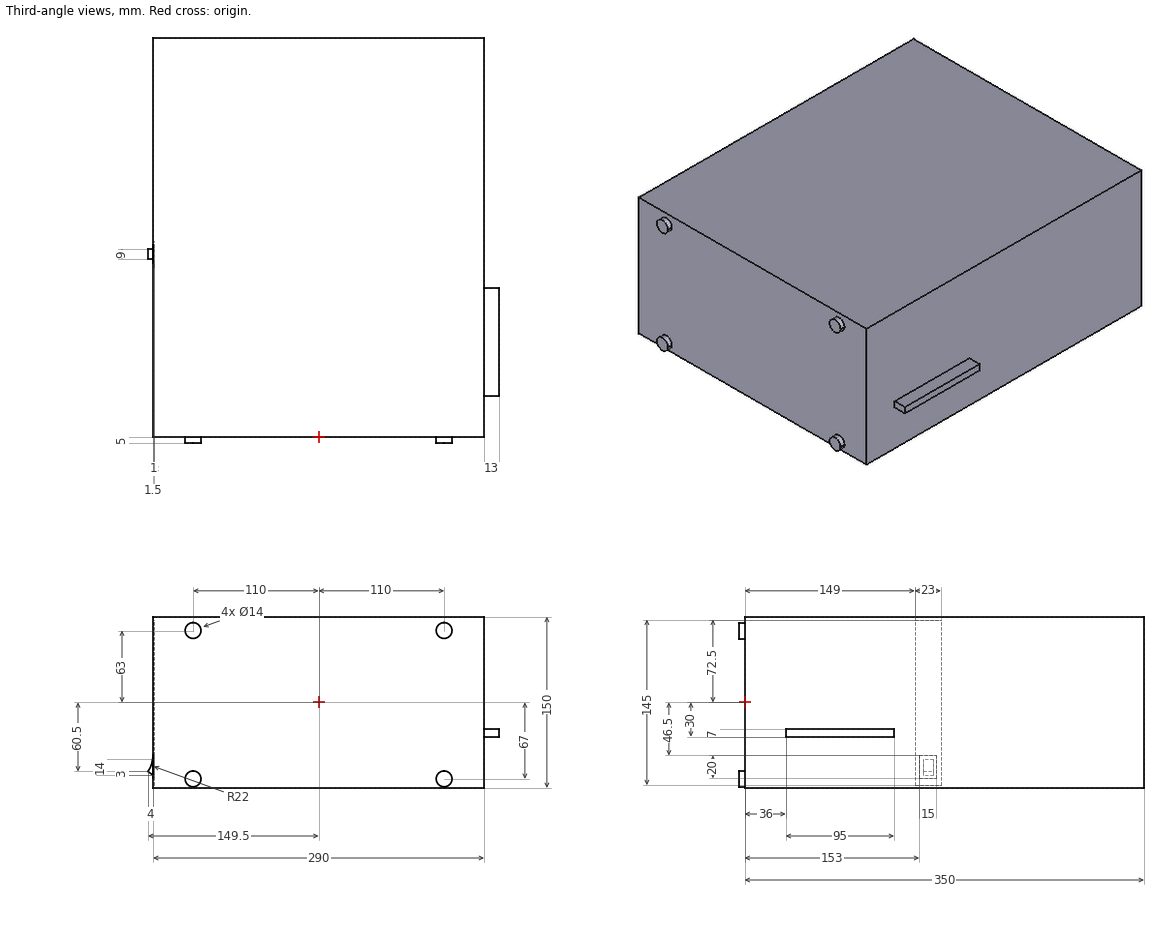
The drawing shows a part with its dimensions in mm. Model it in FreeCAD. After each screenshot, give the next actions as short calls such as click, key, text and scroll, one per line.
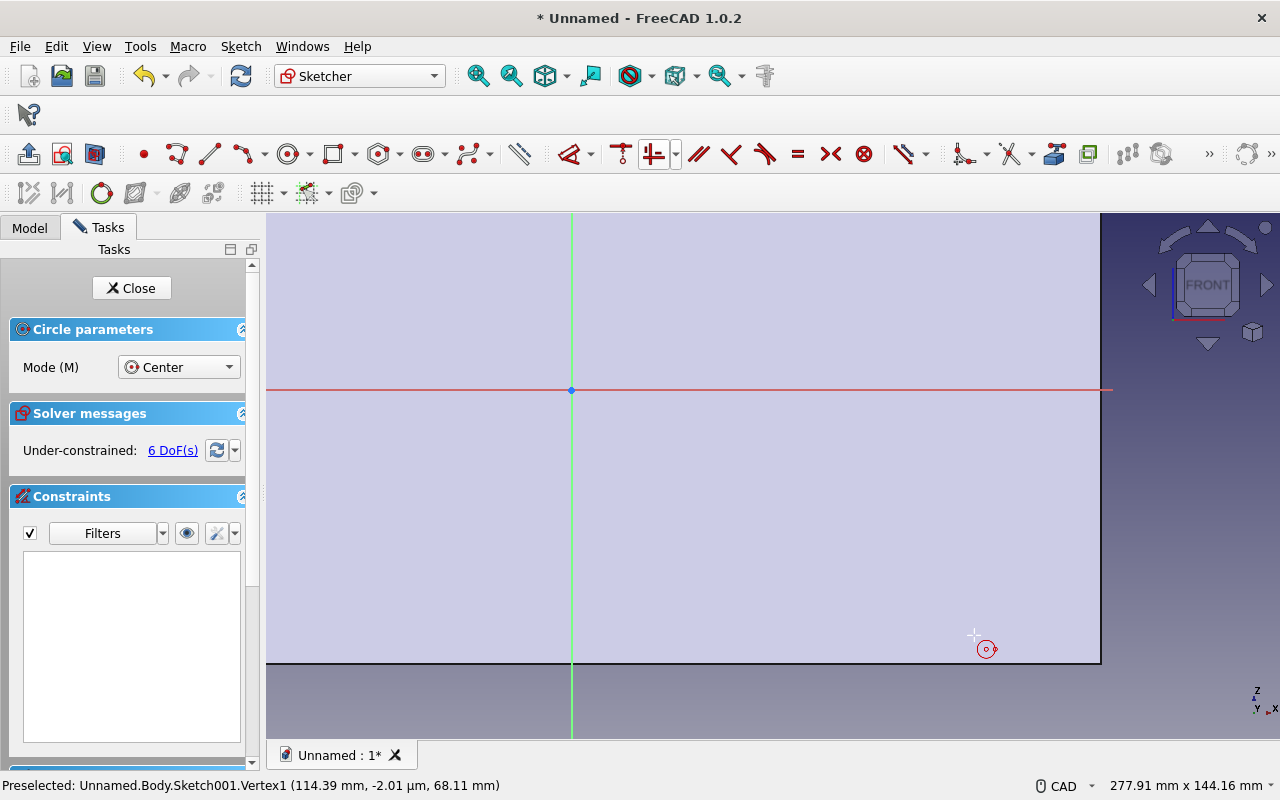
click(973, 635)
click(991, 617)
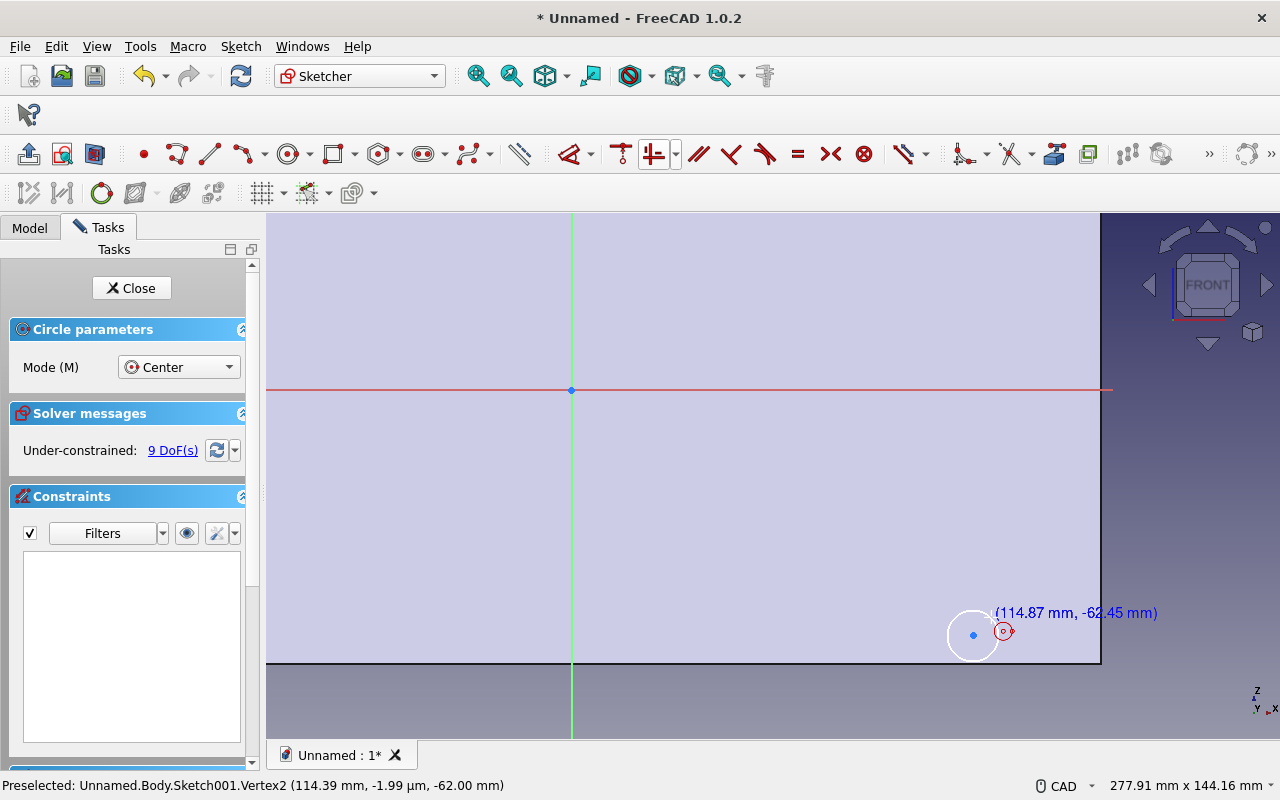
scroll(974, 636, down, 2)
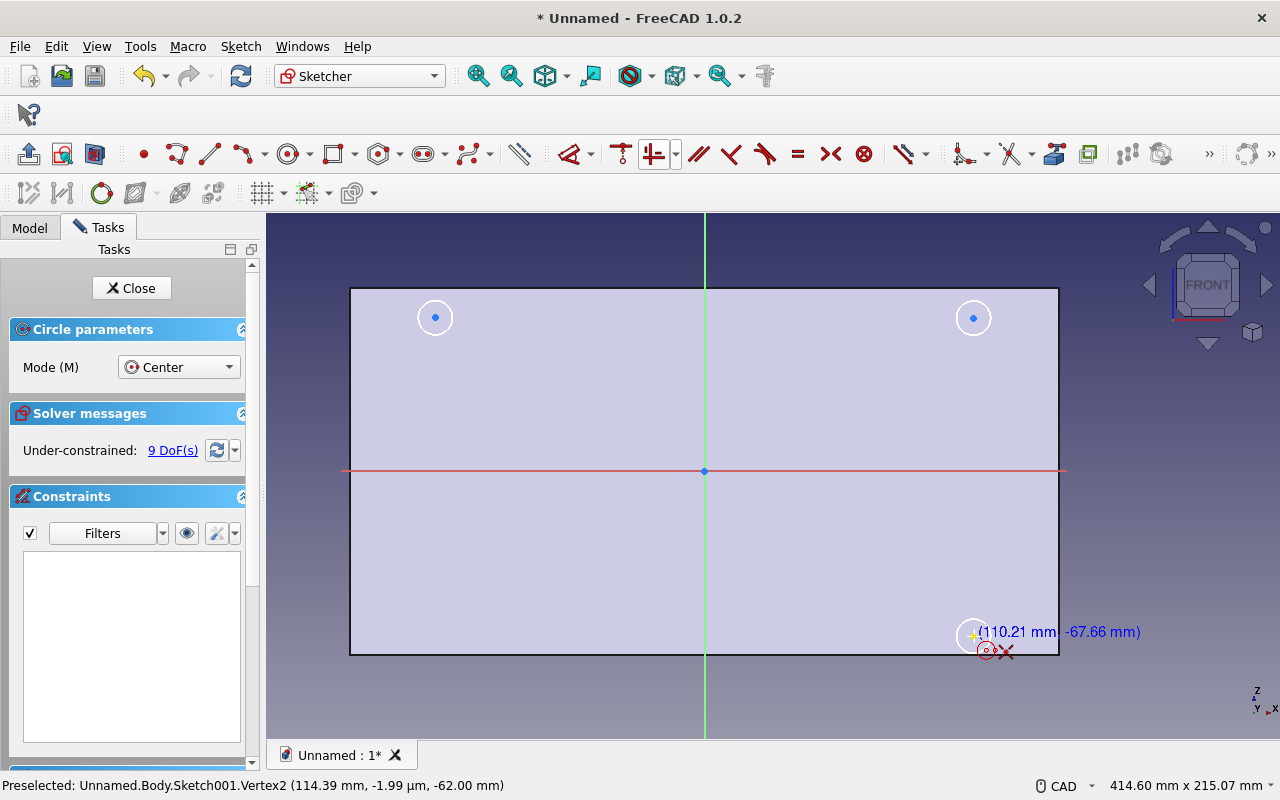
scroll(436, 635, up, 2)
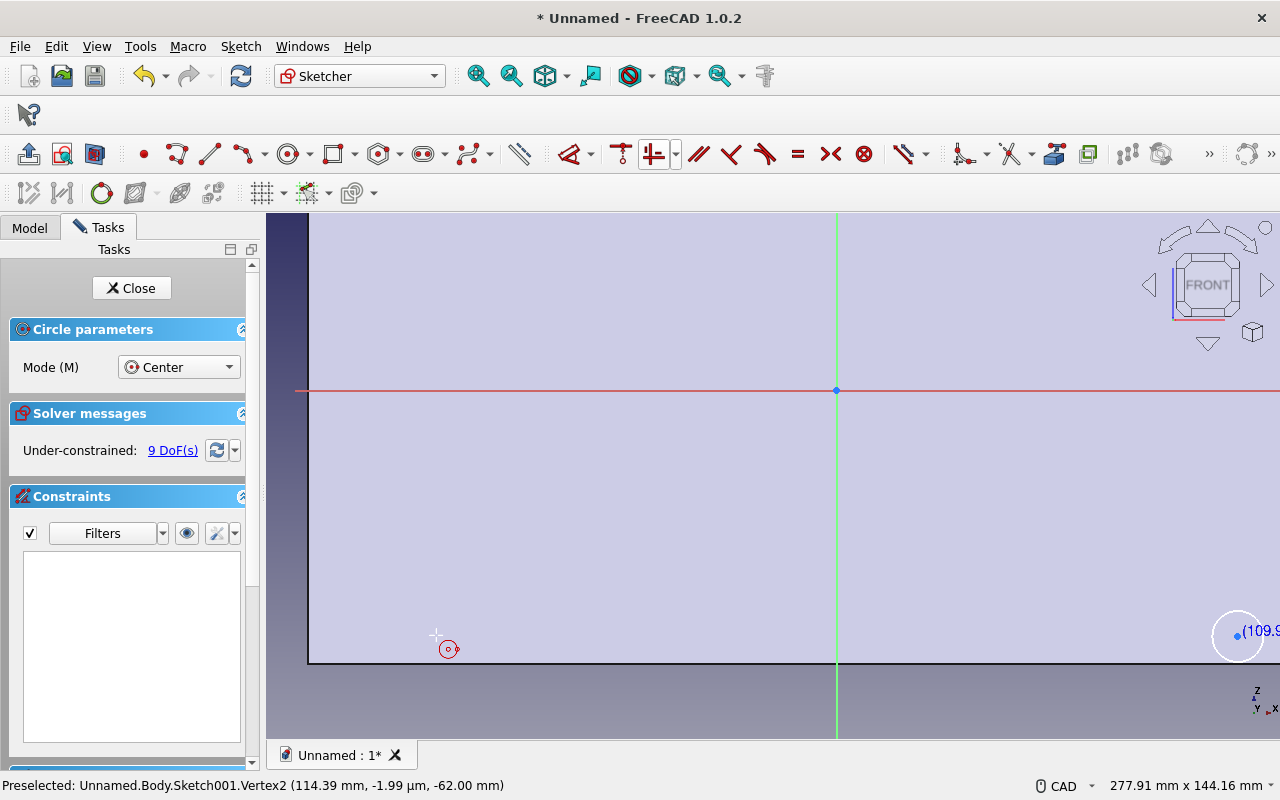
click(435, 635)
click(453, 617)
key(Escape)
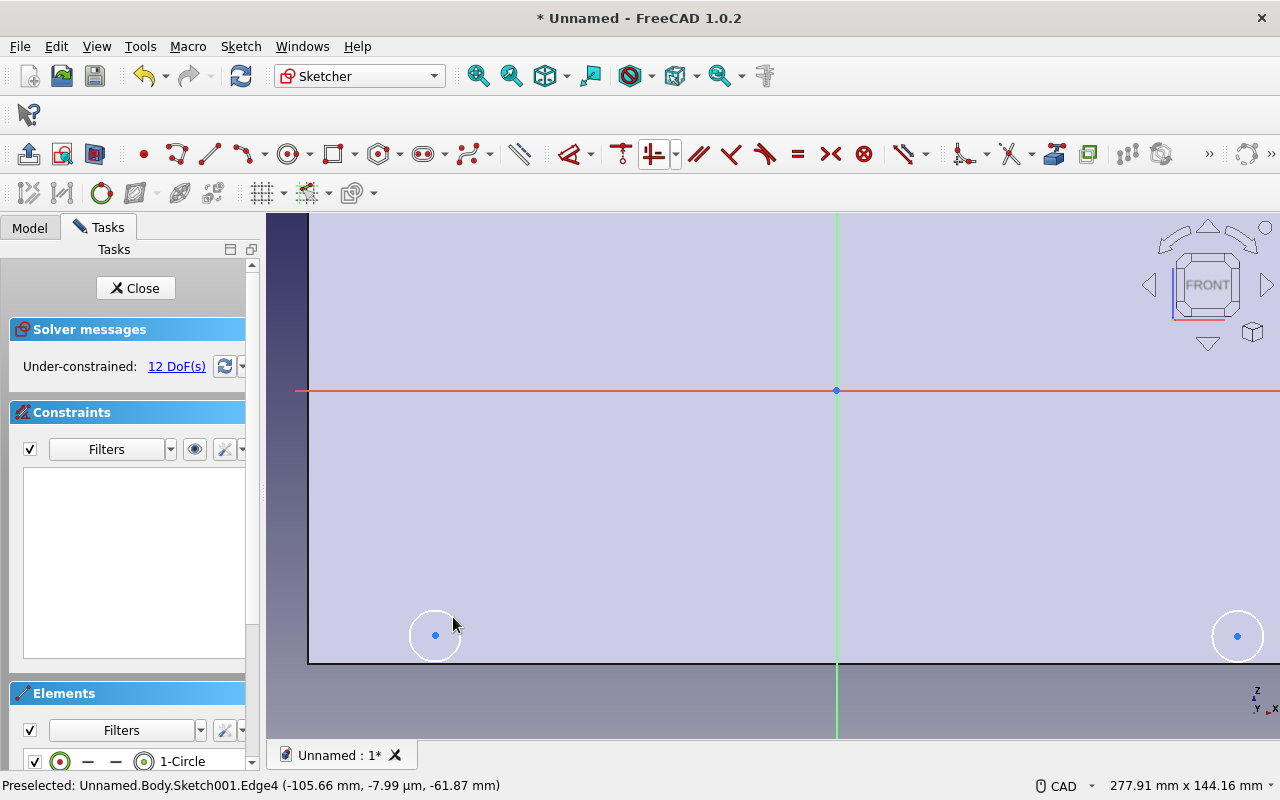
scroll(436, 635, down, 2)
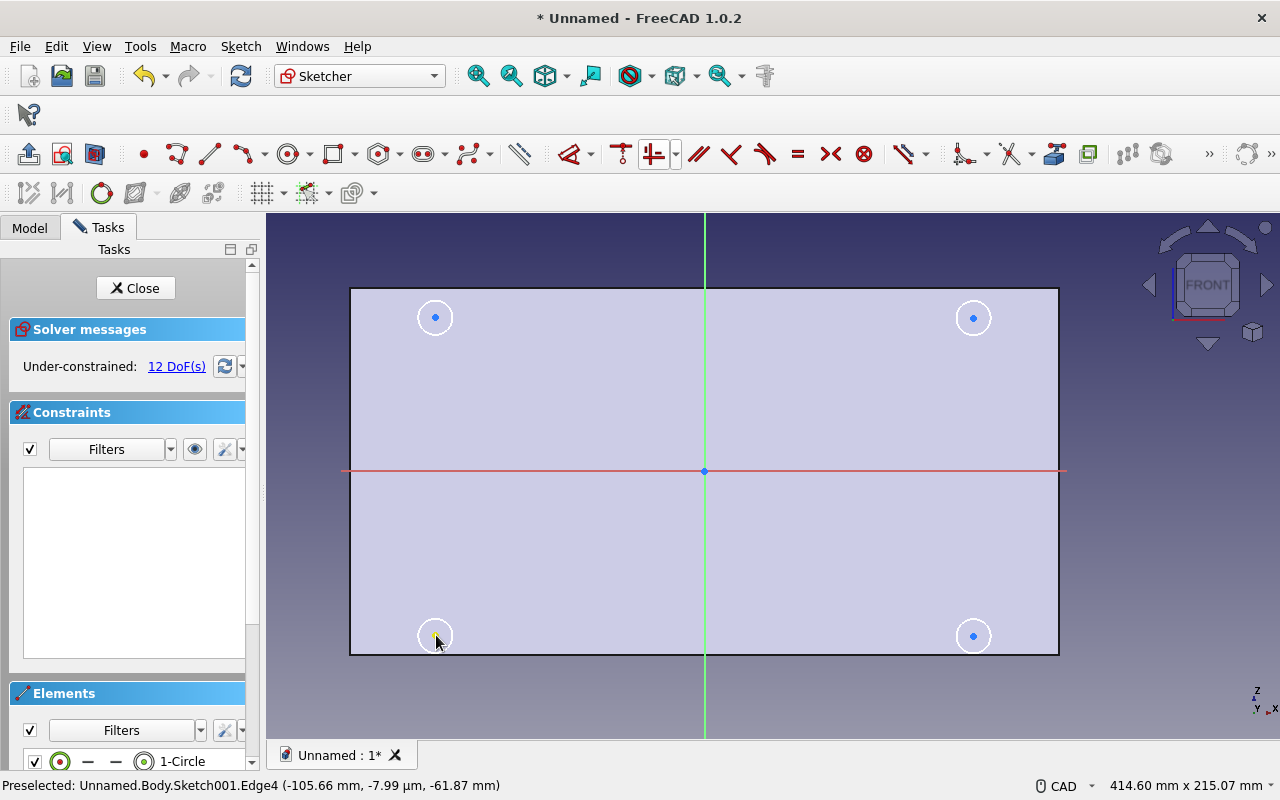
click(447, 306)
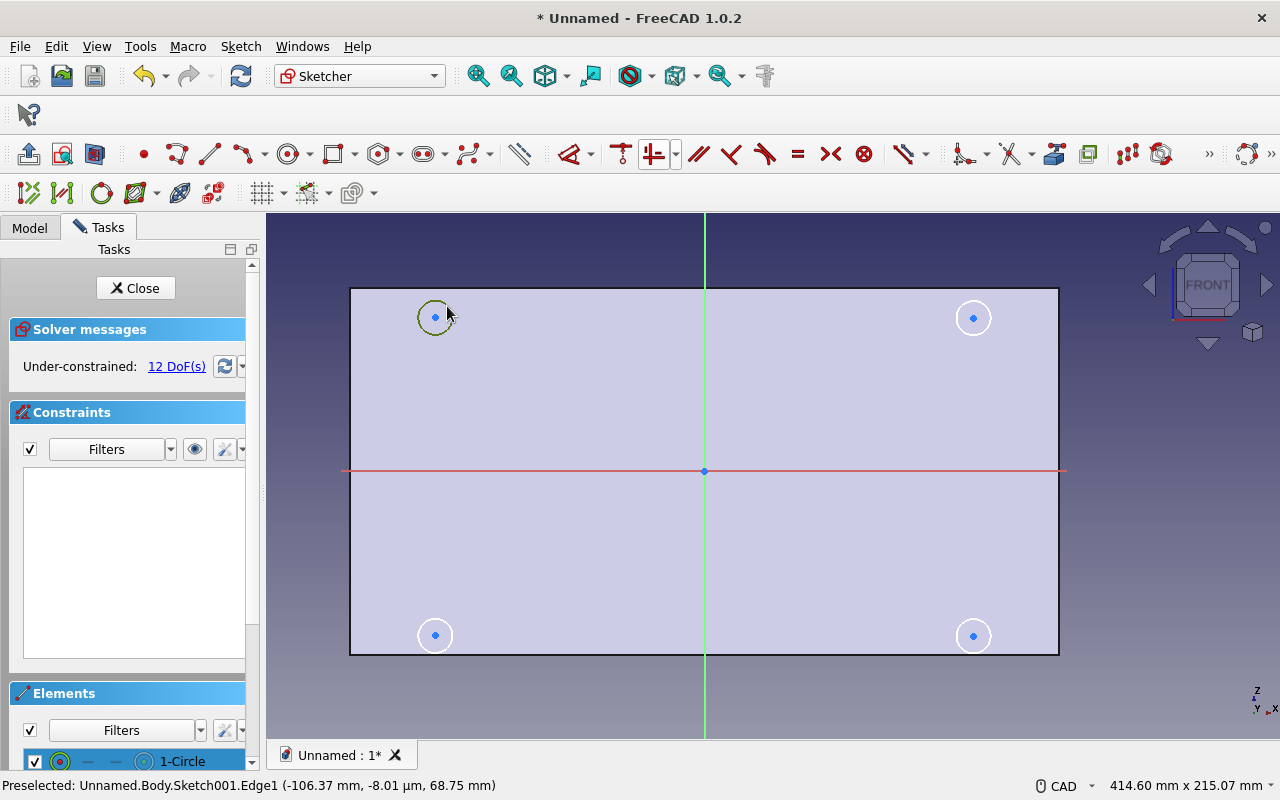
click(986, 306)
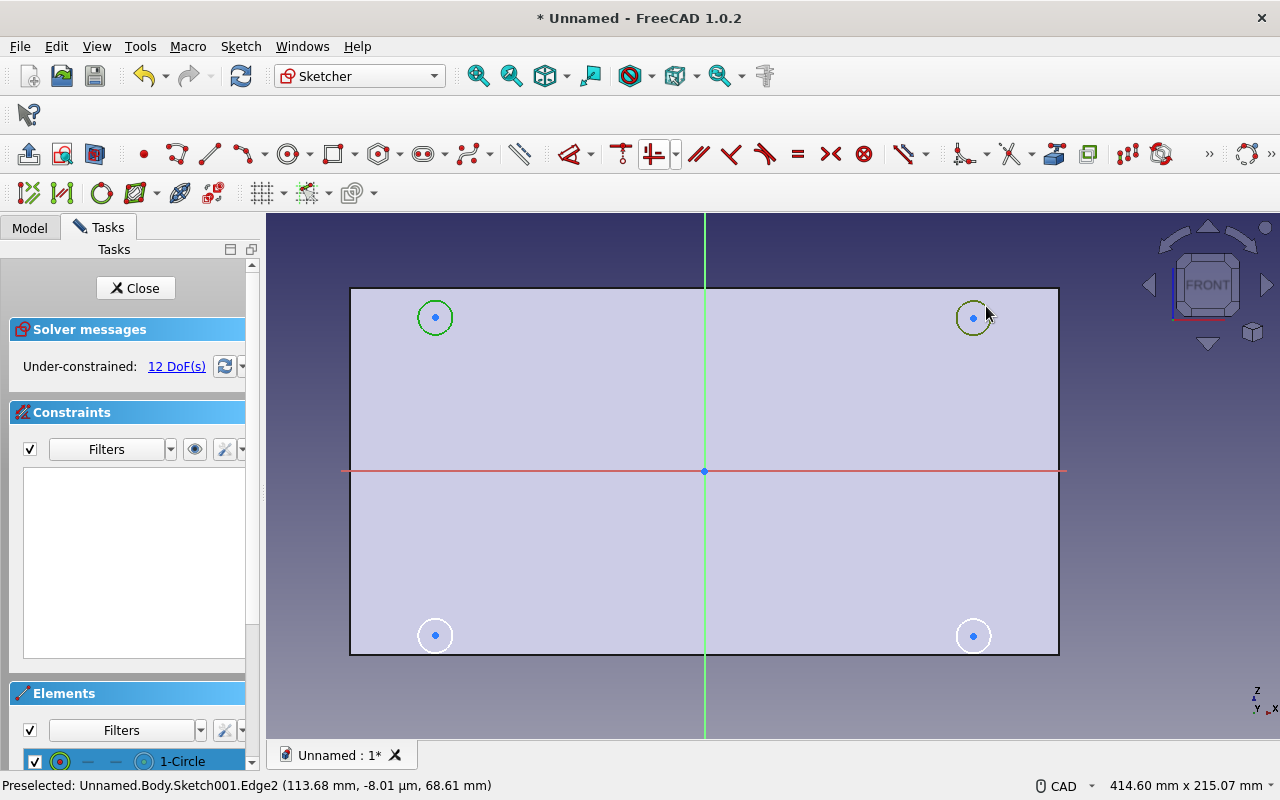
click(986, 624)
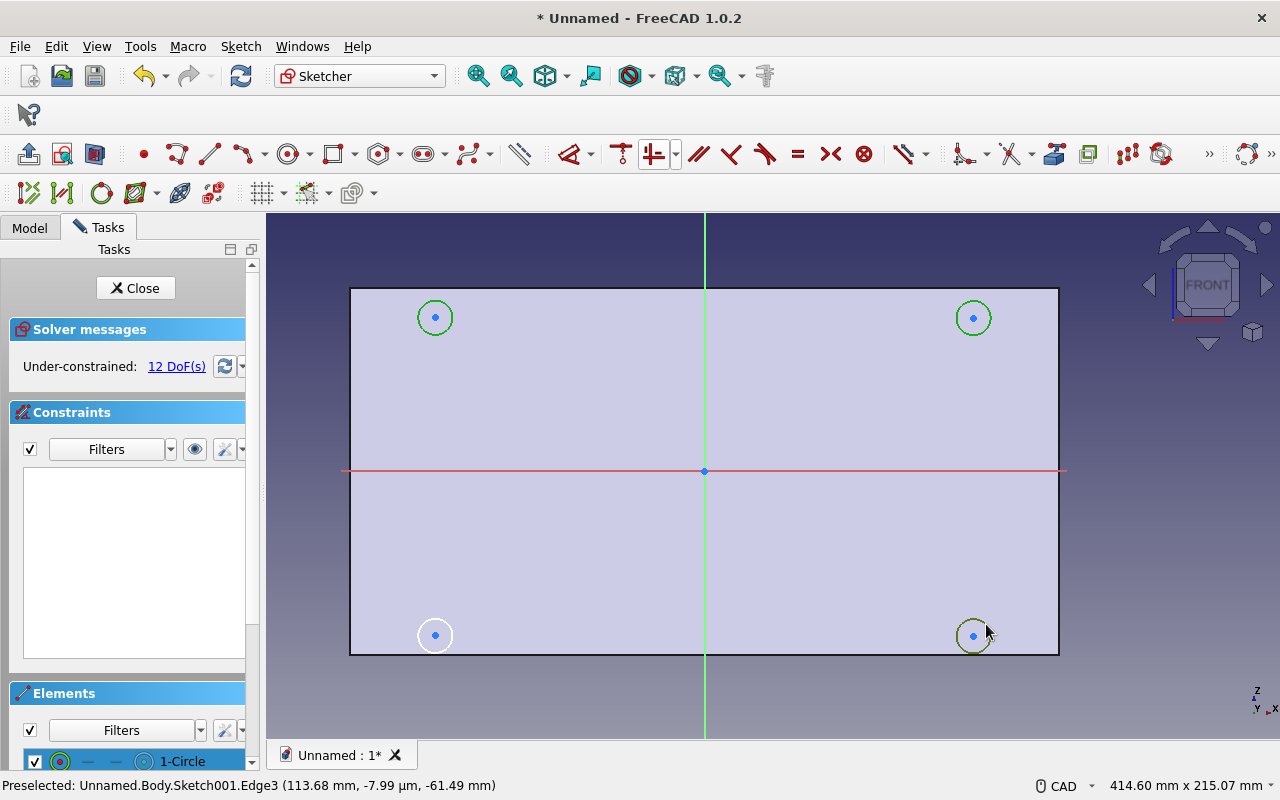
click(447, 624)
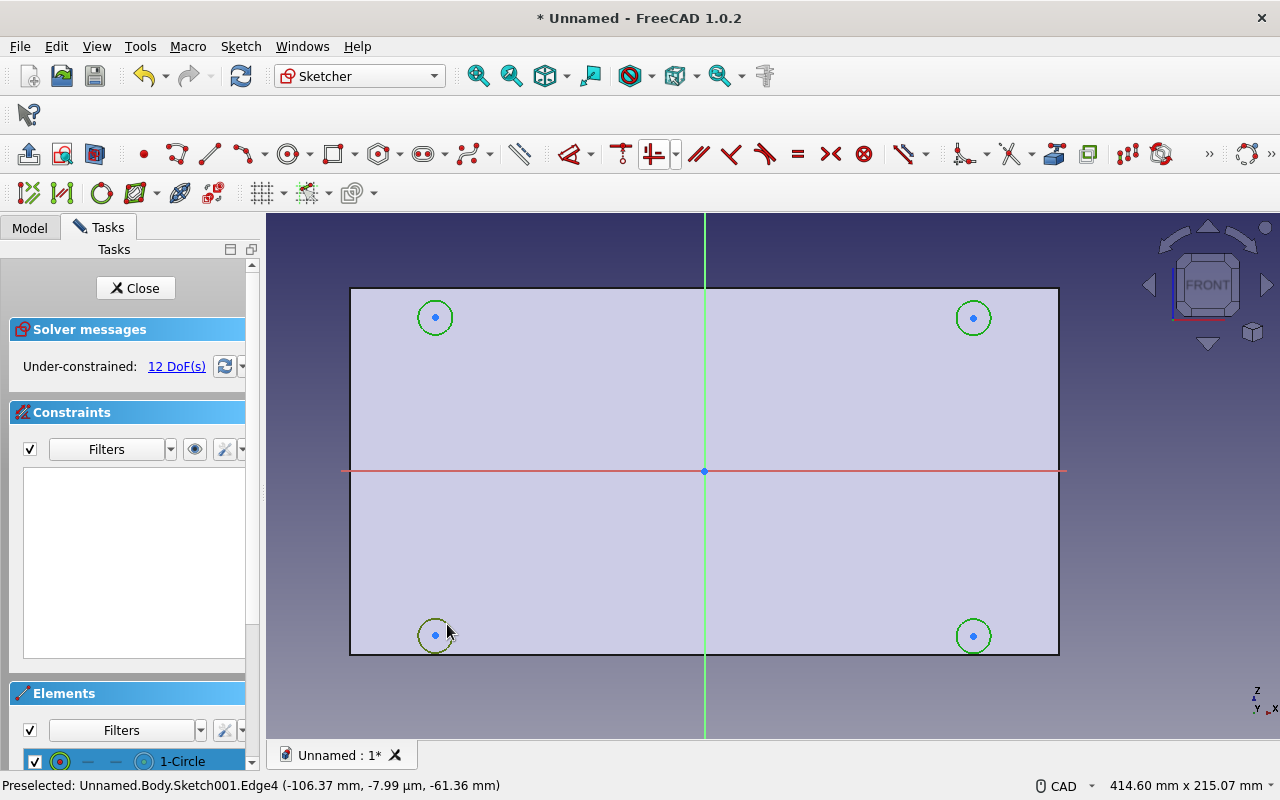
click(798, 154)